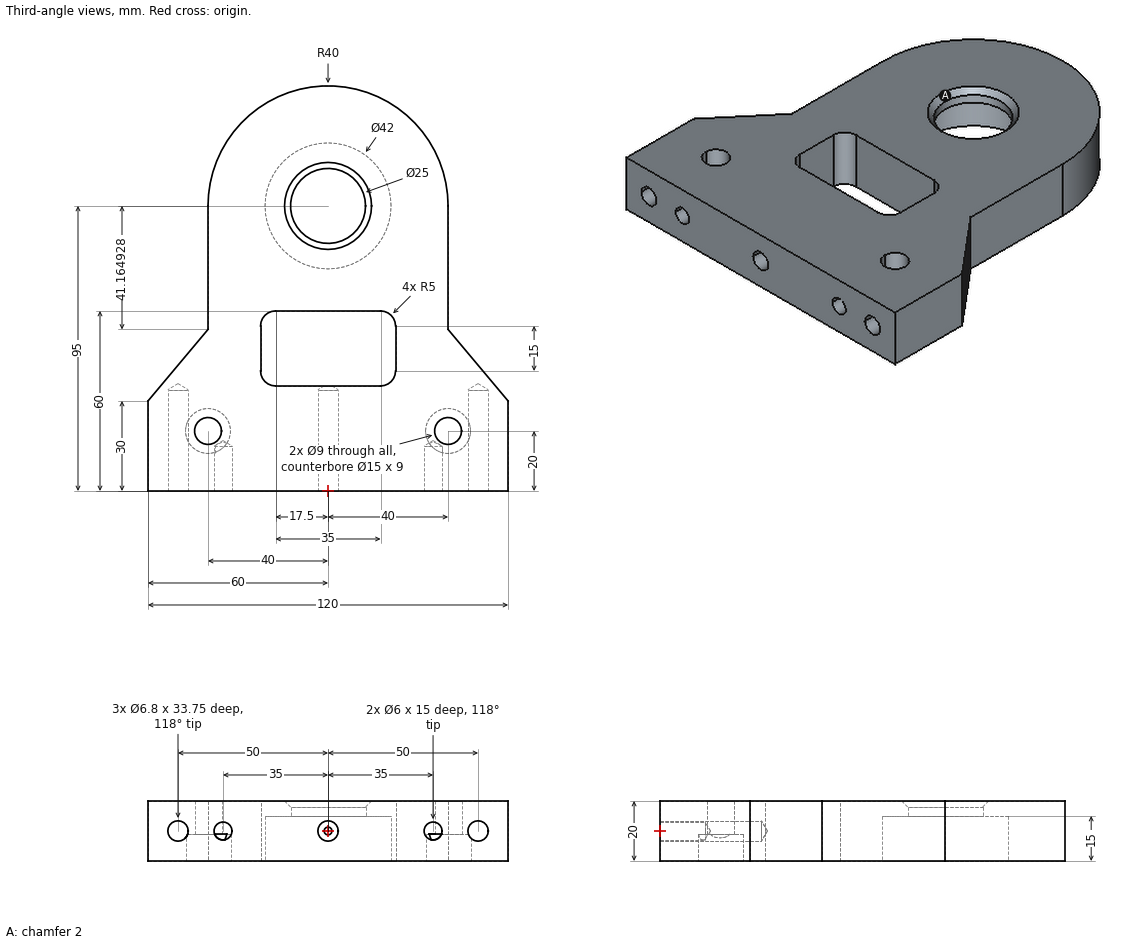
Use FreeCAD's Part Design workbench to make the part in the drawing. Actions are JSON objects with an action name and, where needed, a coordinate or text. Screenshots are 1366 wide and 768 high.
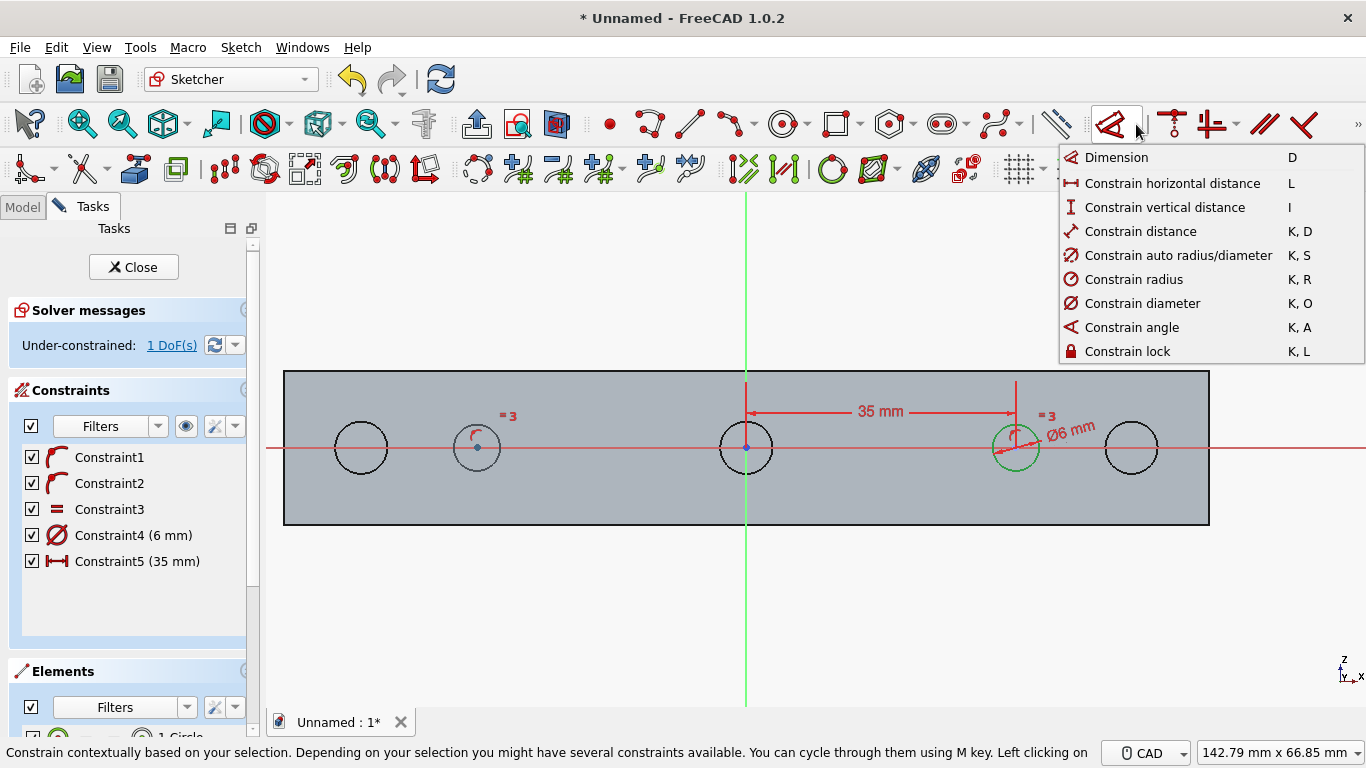
{"action": "left_click", "coordinate": [1212, 183]}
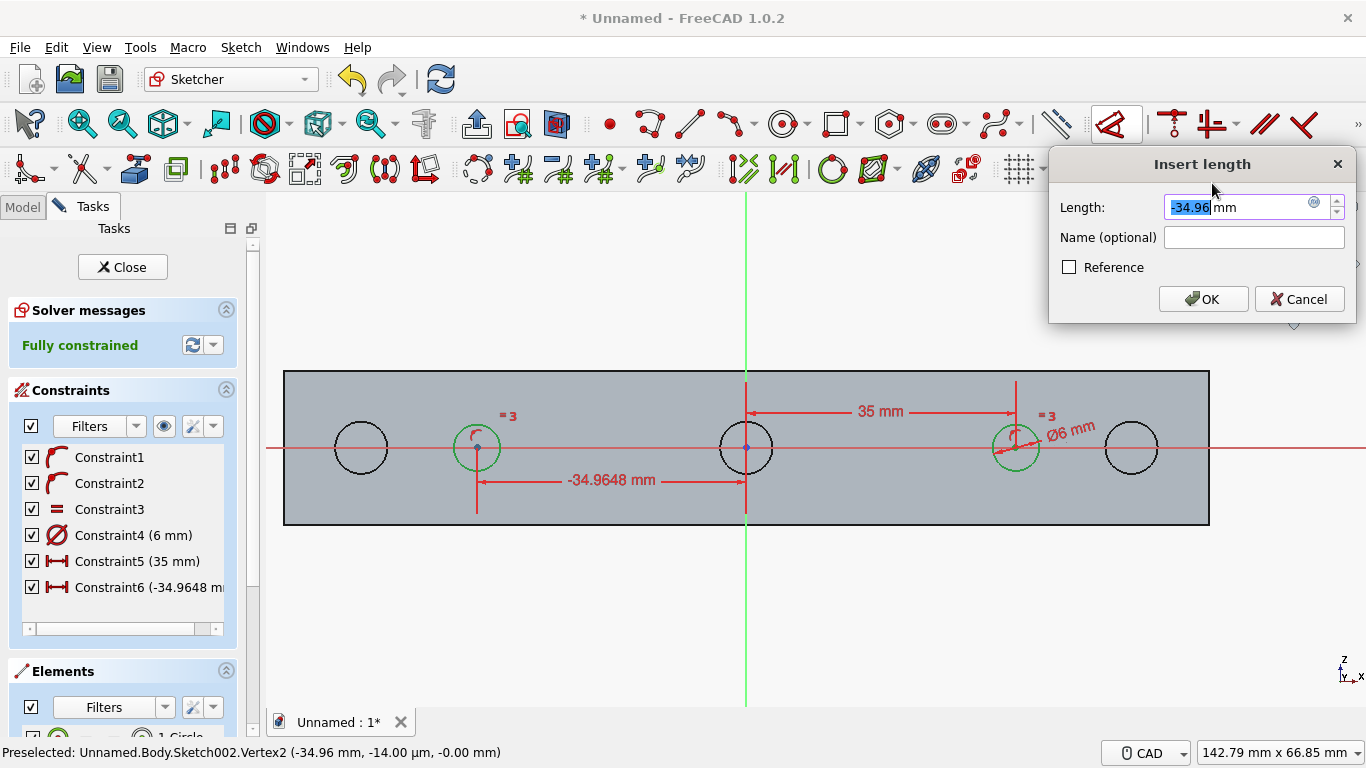
{"action": "type", "text": "-35"}
{"action": "key", "text": "Return"}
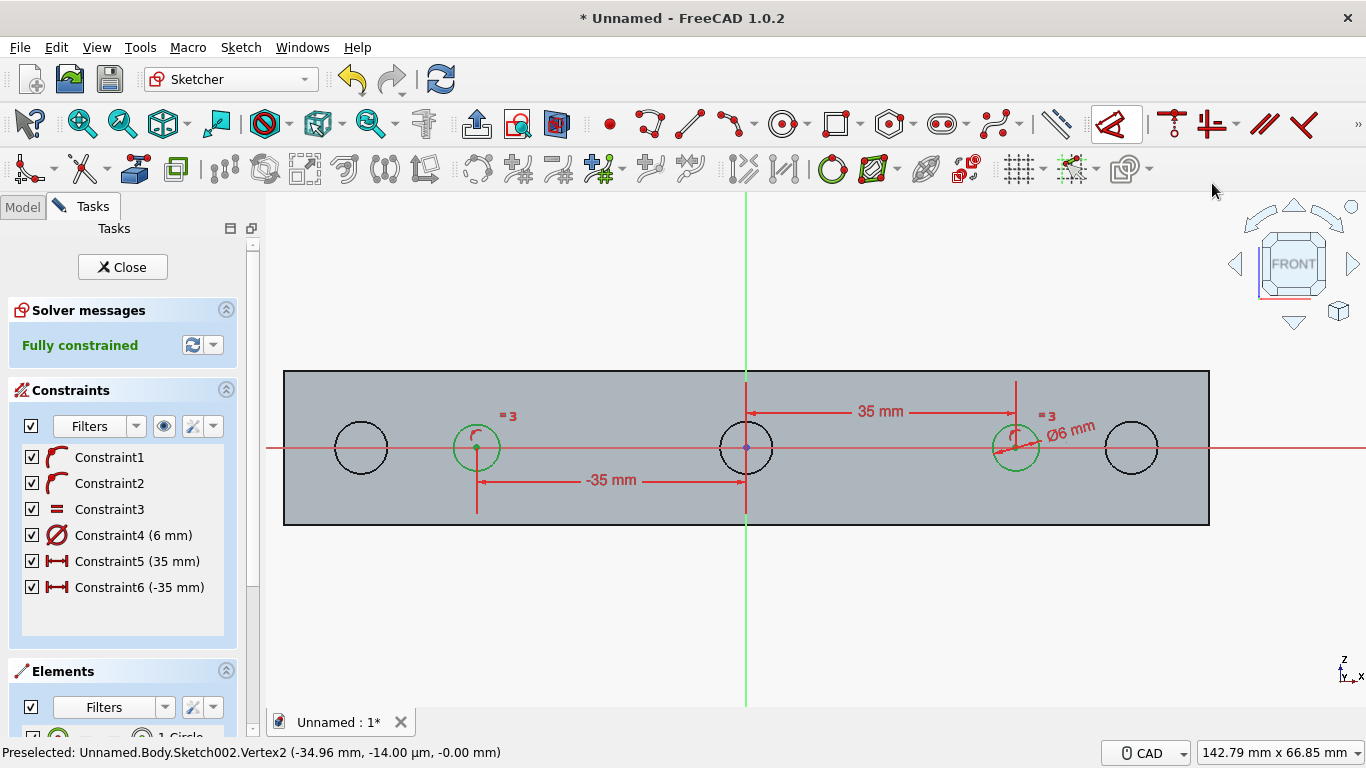
{"action": "left_click", "coordinate": [123, 267]}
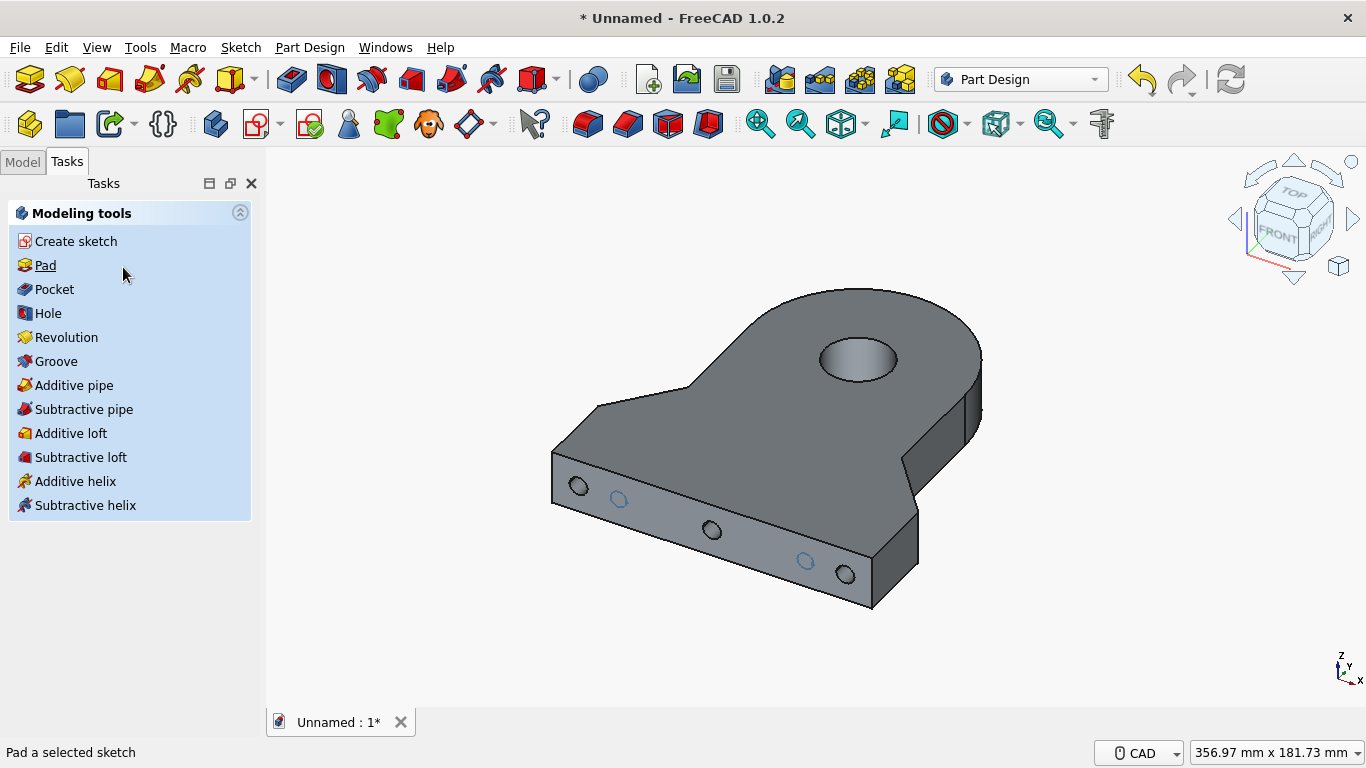
{"action": "left_click", "coordinate": [332, 80]}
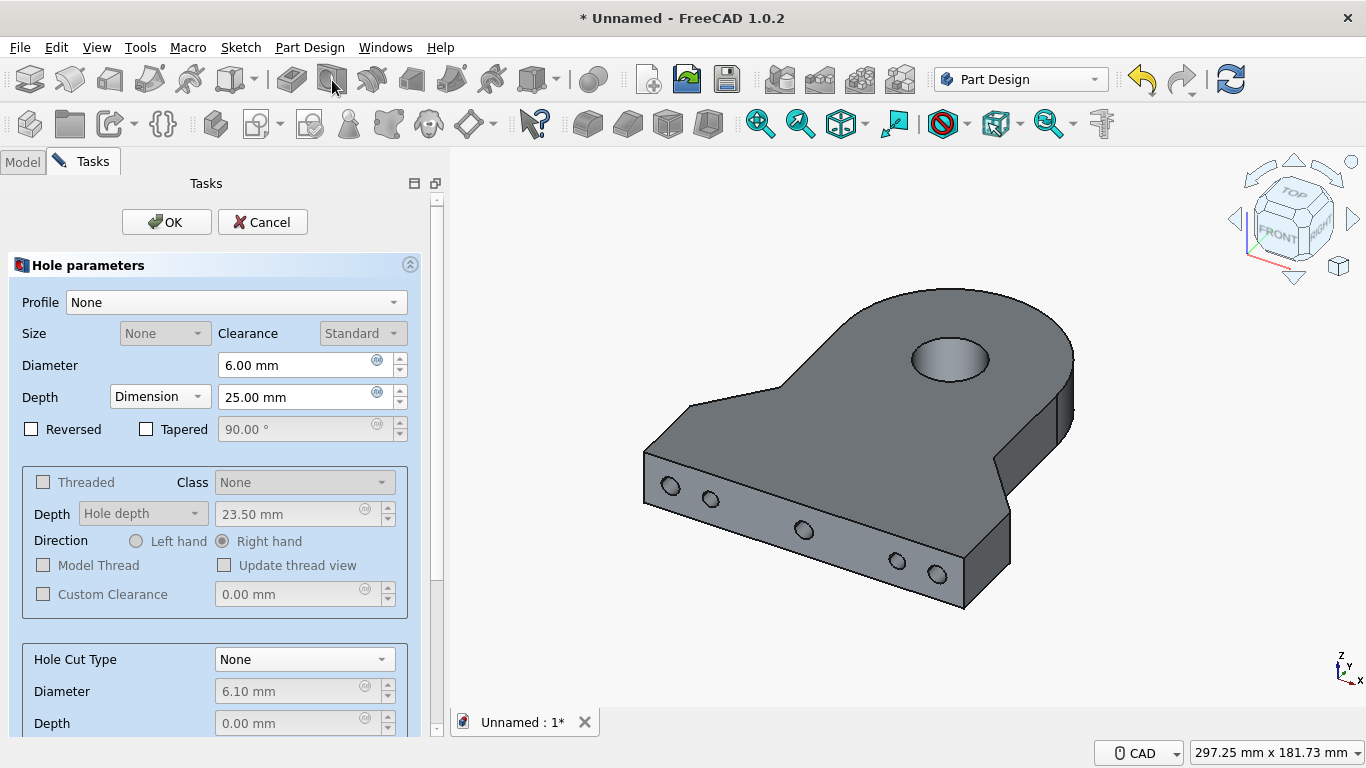
{"action": "triple_click", "coordinate": [305, 365]}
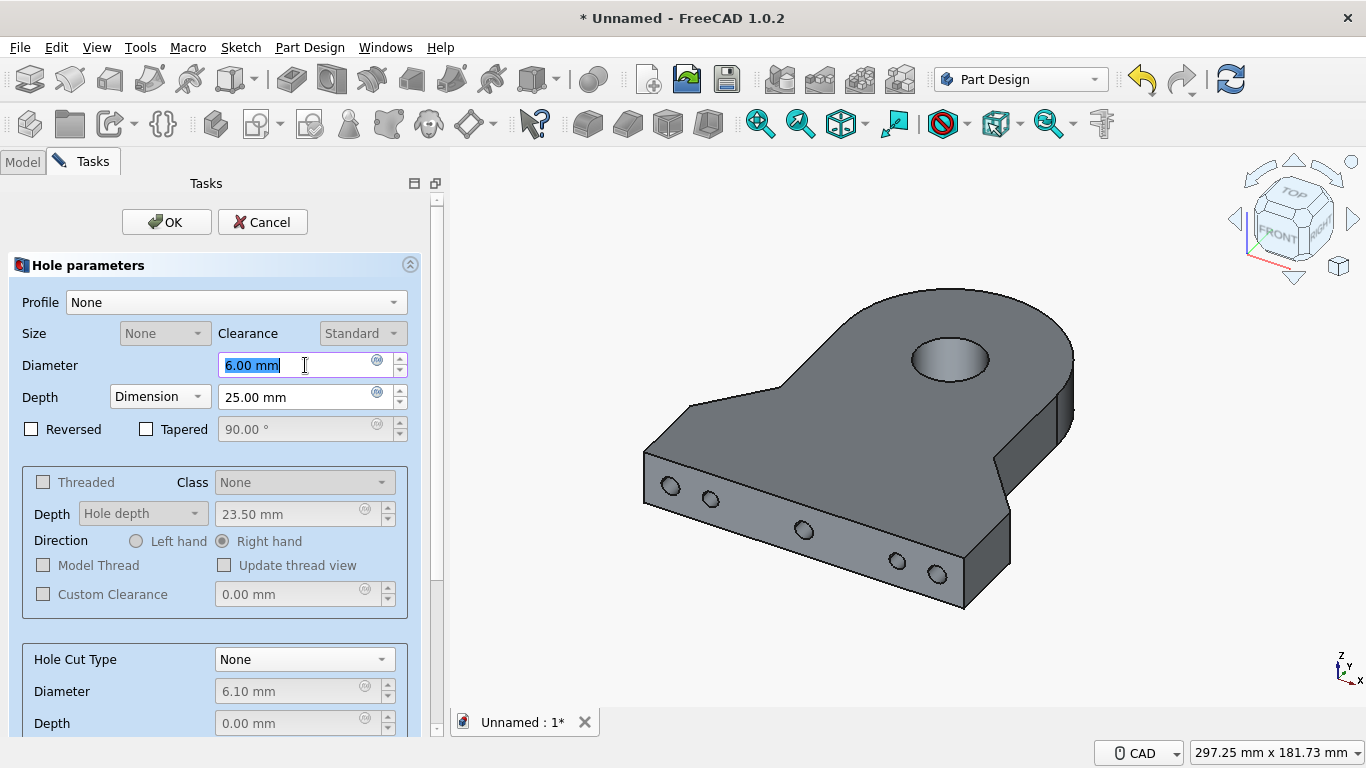
{"action": "type", "text": "6"}
{"action": "key", "text": "Tab"}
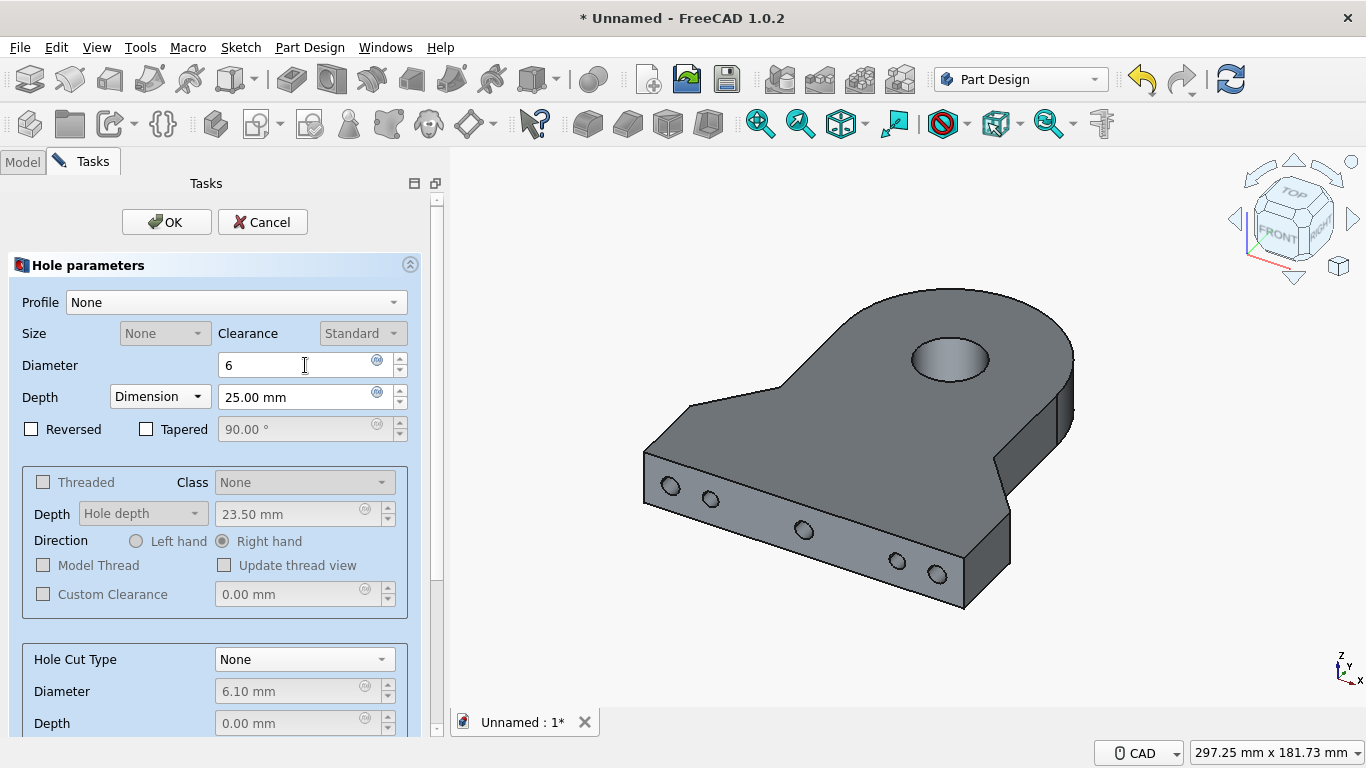
{"action": "triple_click", "coordinate": [305, 397]}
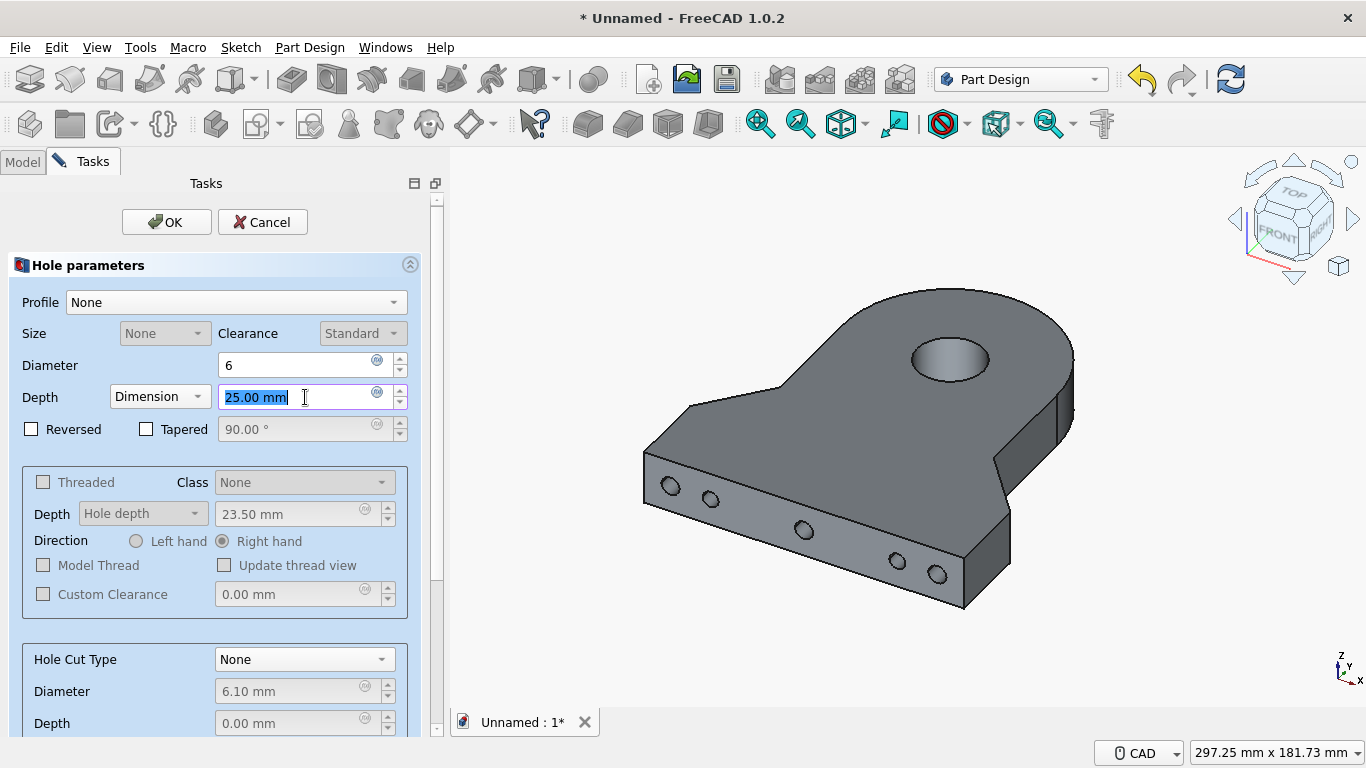
{"action": "type", "text": "15"}
{"action": "key", "text": "Tab"}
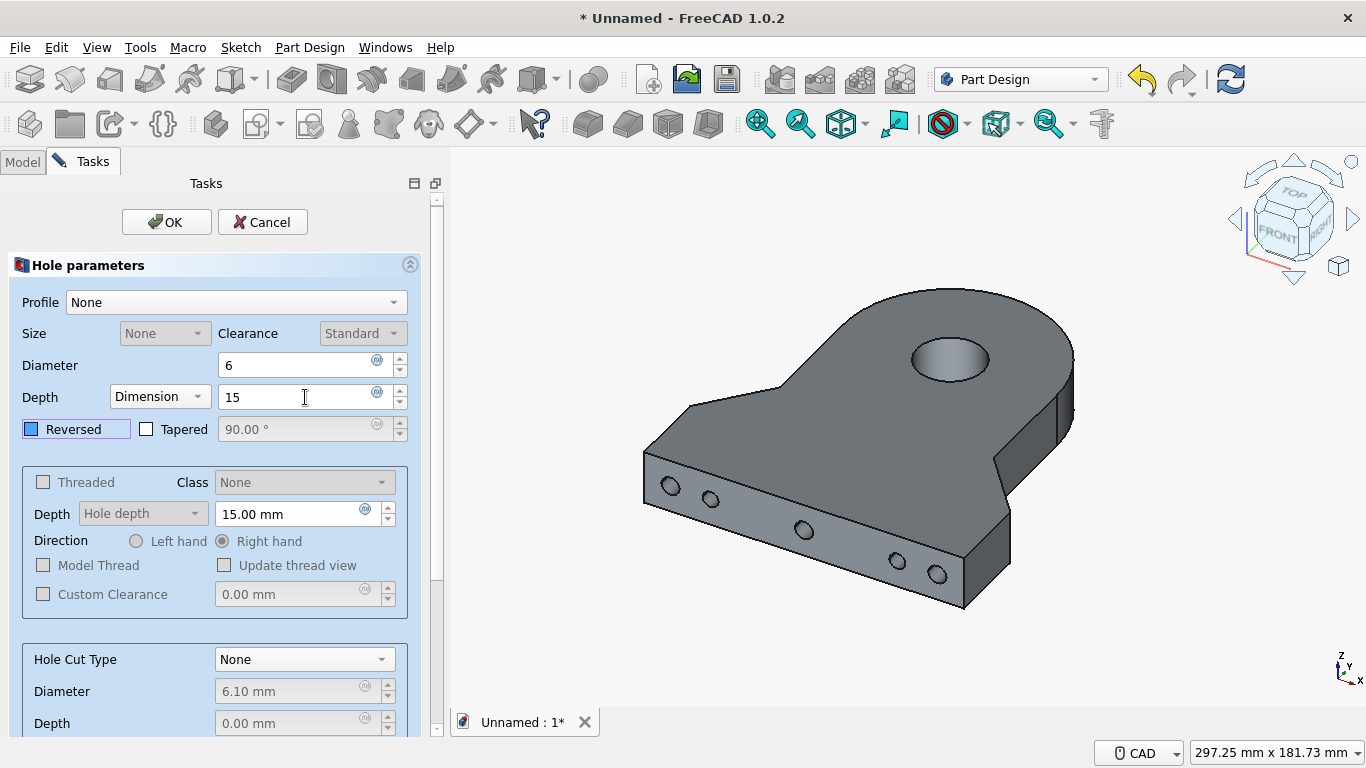
{"action": "left_click", "coordinate": [167, 222]}